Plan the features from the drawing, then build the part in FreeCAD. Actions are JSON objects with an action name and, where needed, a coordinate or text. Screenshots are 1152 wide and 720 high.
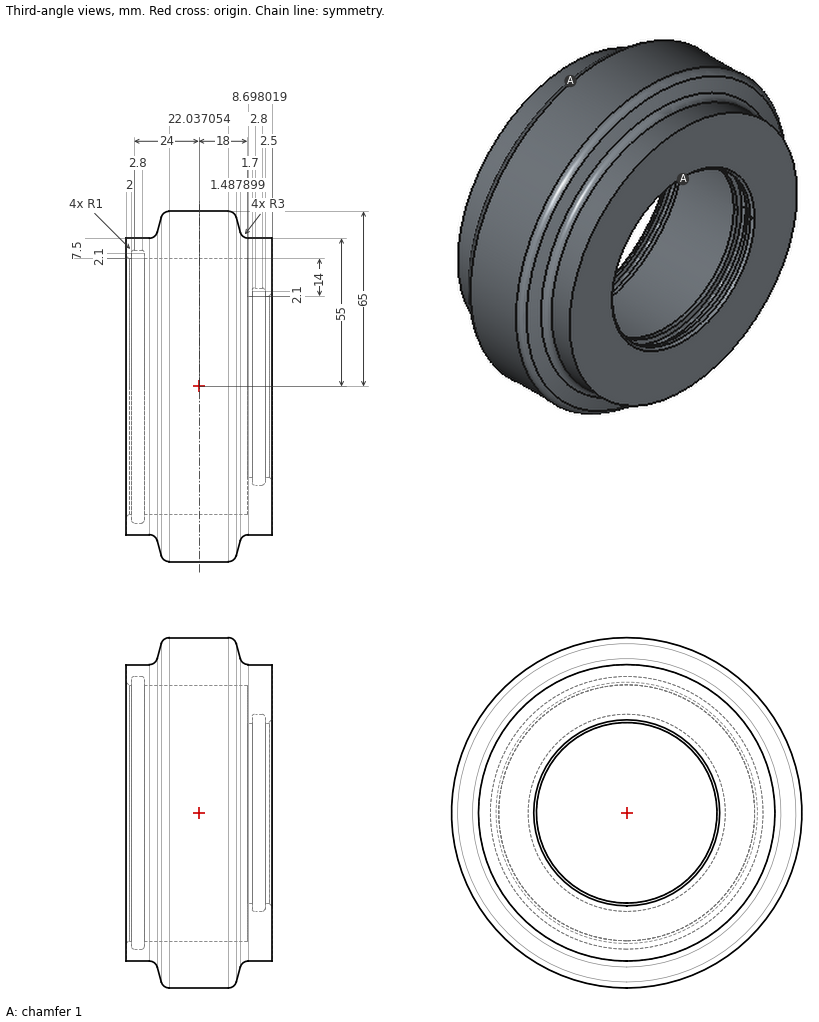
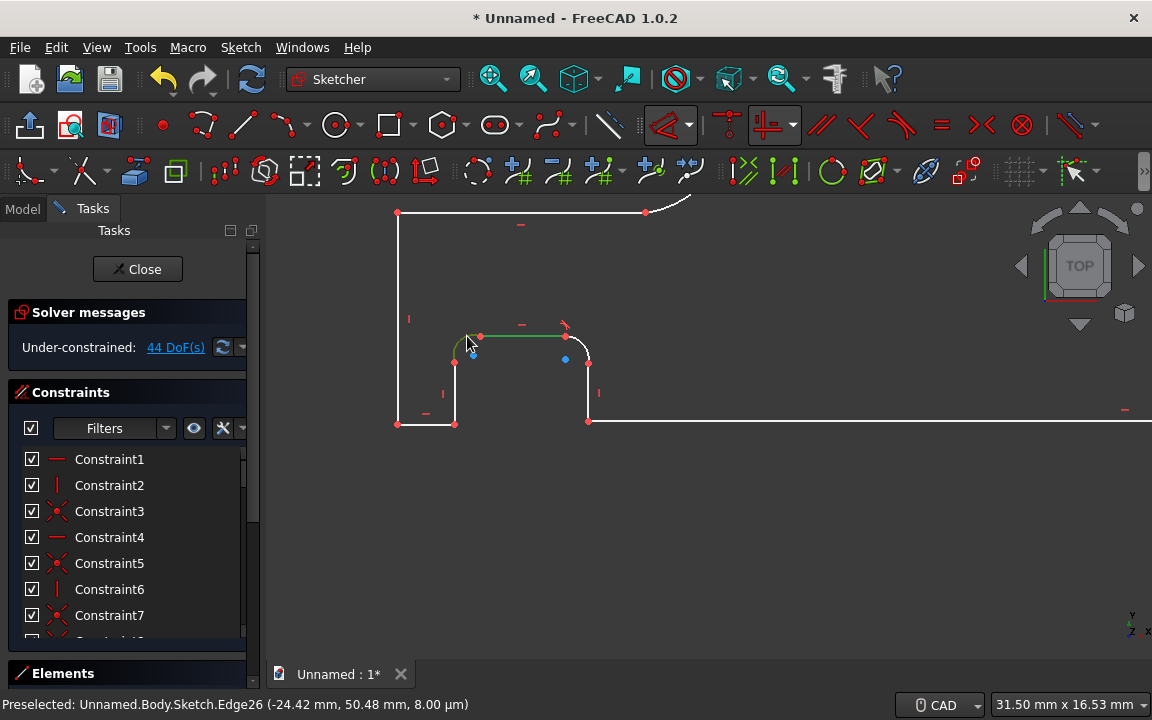
{"action": "left_click", "coordinate": [902, 126]}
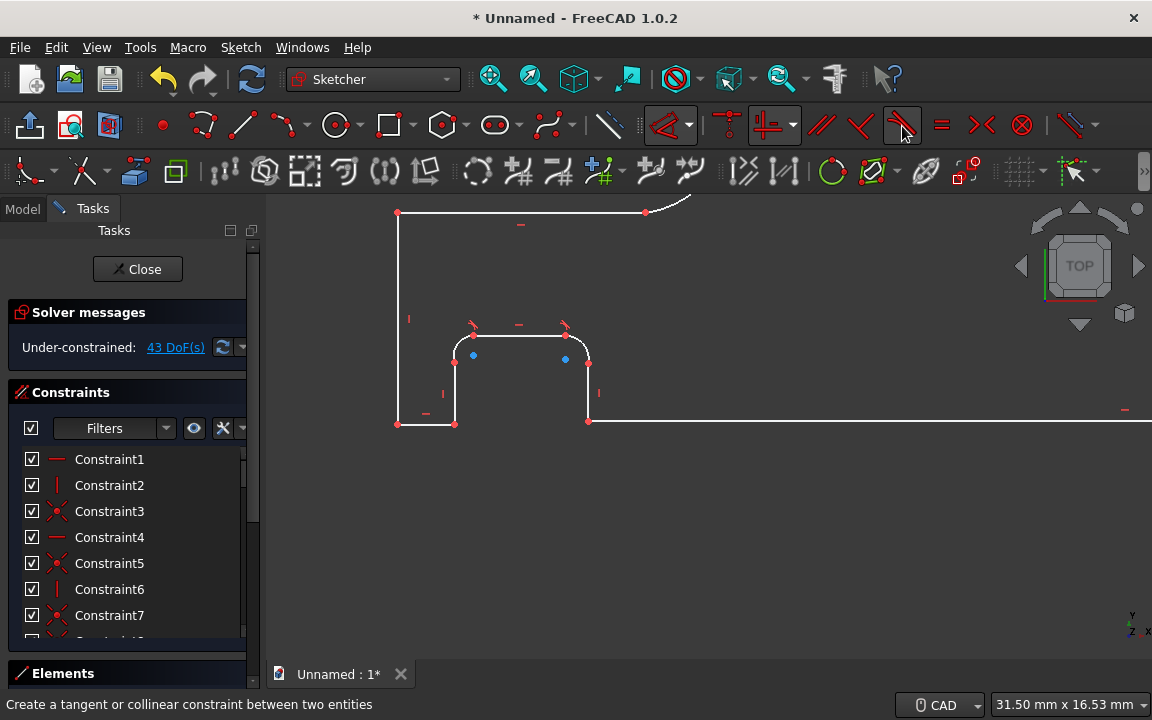
{"action": "left_click", "coordinate": [588, 381]}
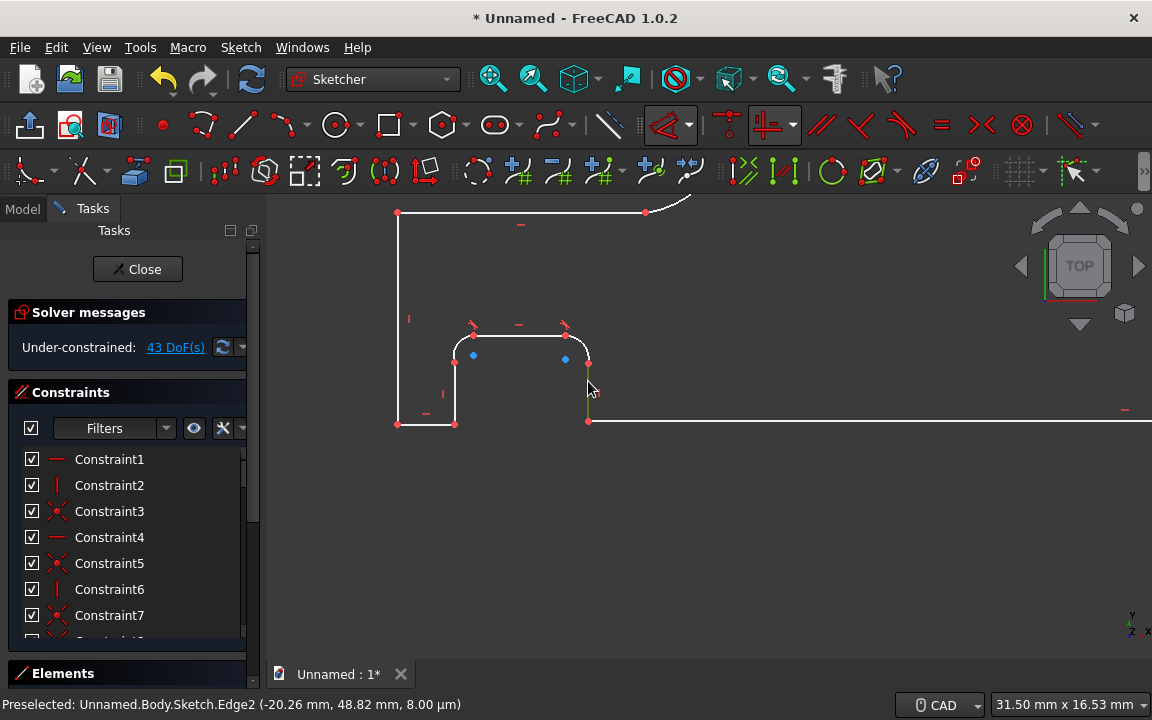
{"action": "left_click", "coordinate": [587, 352]}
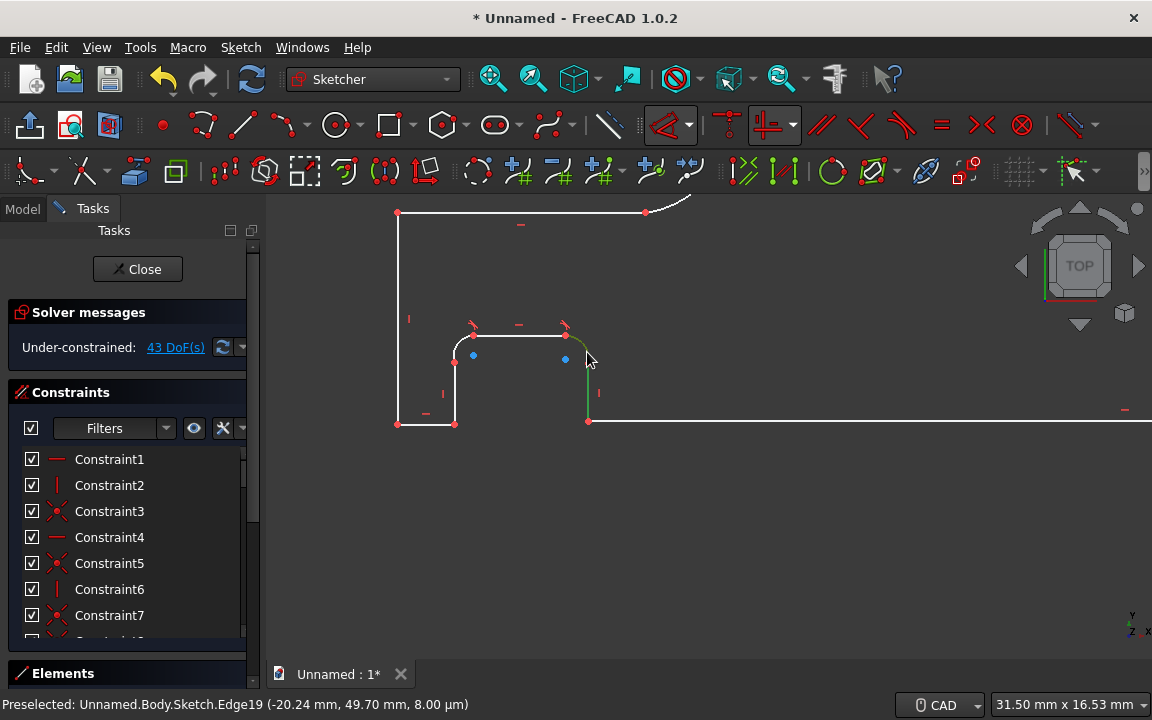
{"action": "key", "text": "t"}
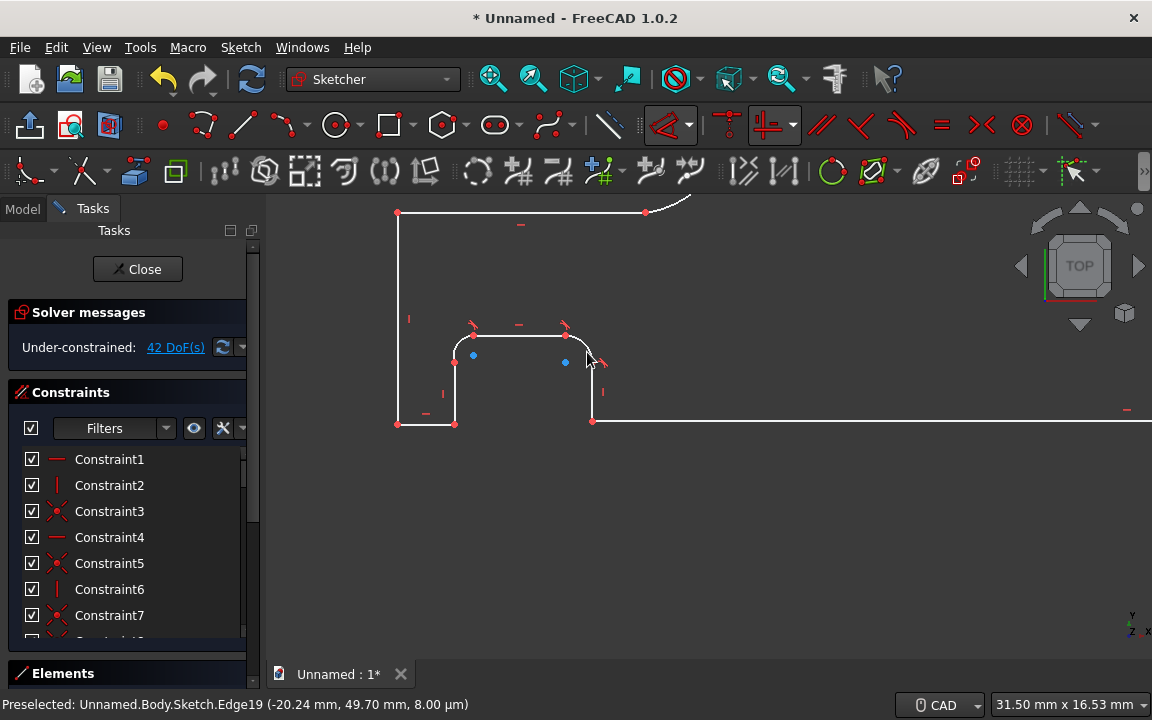
{"action": "scroll", "coordinate": [538, 344], "scroll_direction": "down", "scroll_amount": 9}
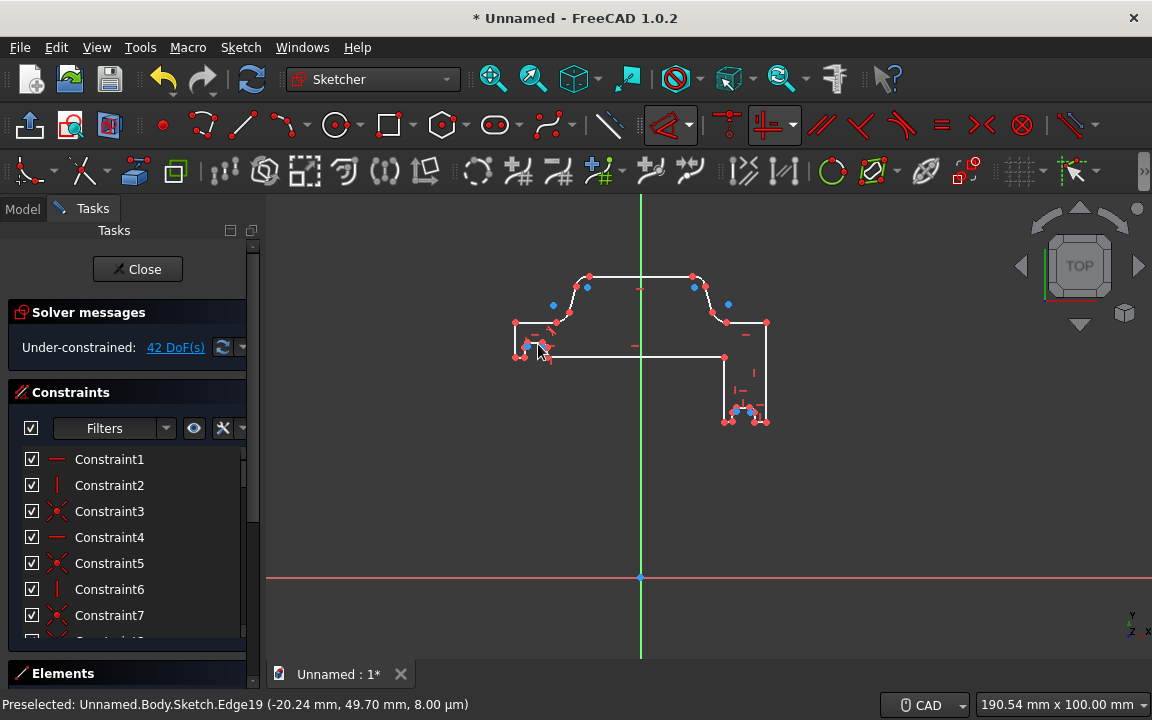
{"action": "scroll", "coordinate": [732, 419], "scroll_direction": "up", "scroll_amount": 8}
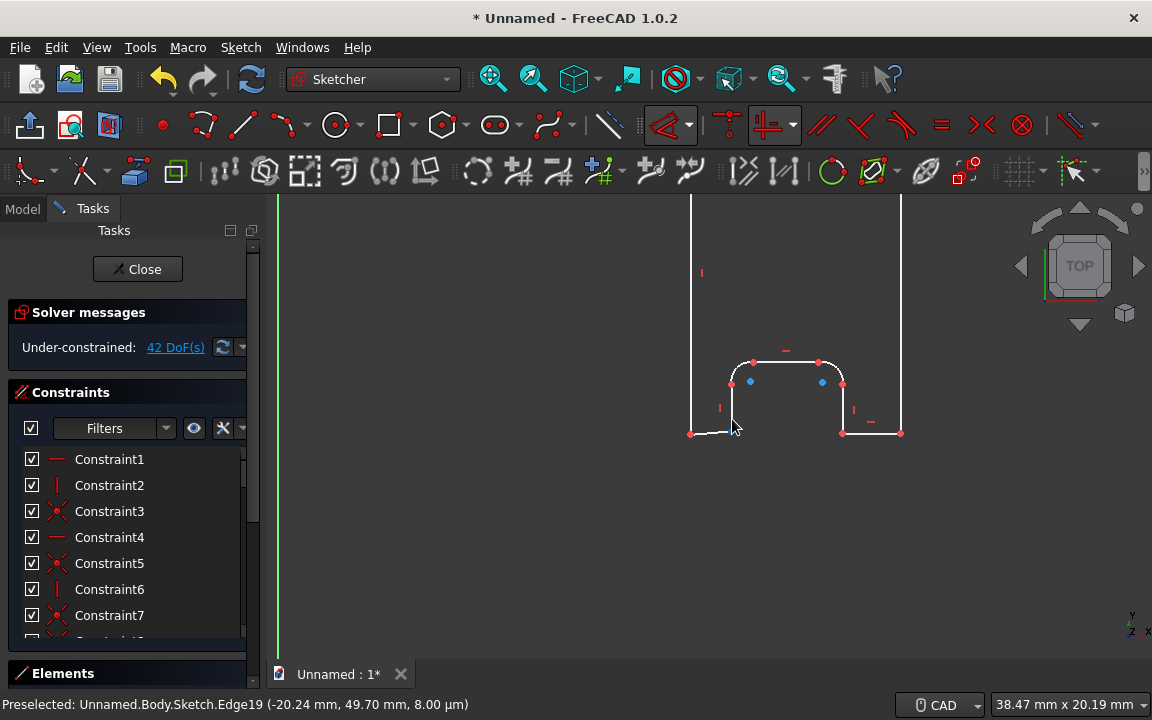
{"action": "left_click", "coordinate": [732, 417]}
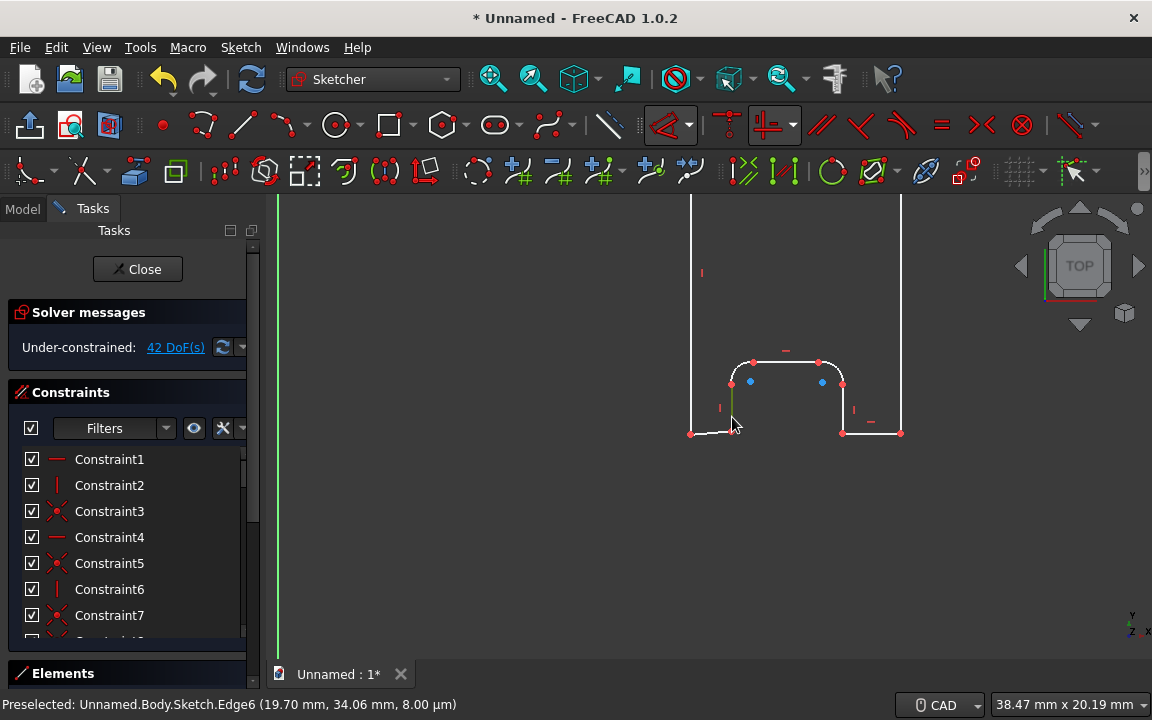
{"action": "scroll", "coordinate": [743, 364], "scroll_direction": "up", "scroll_amount": 2}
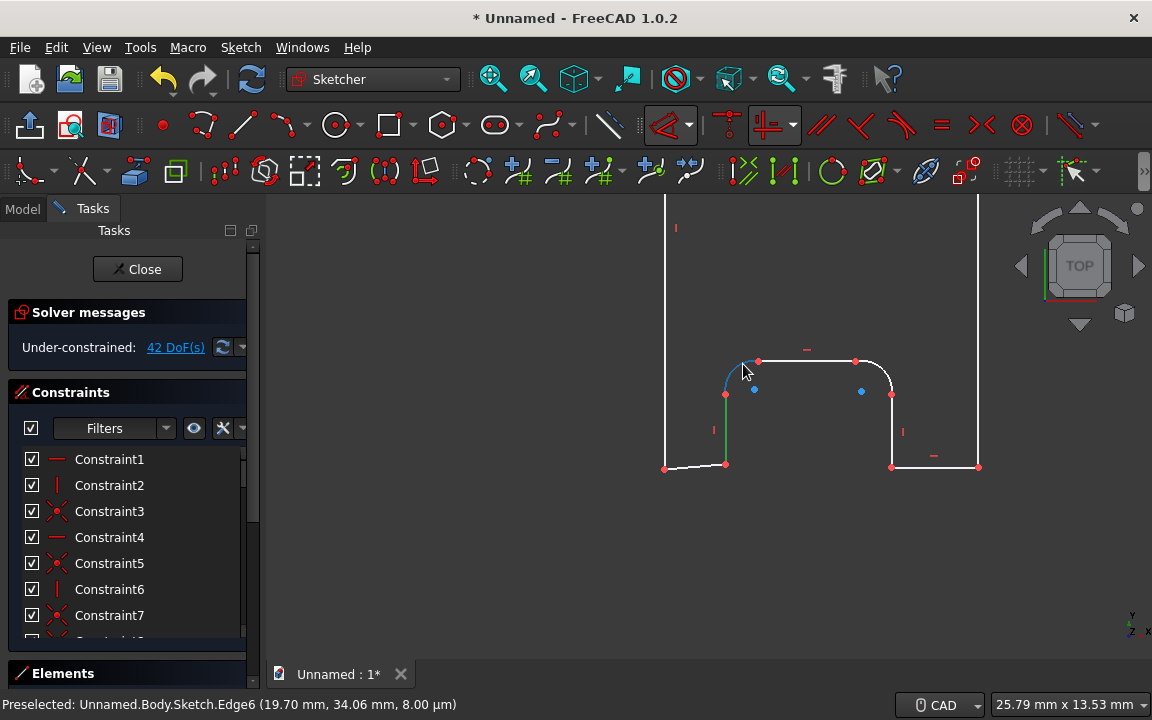
{"action": "left_click", "coordinate": [743, 363]}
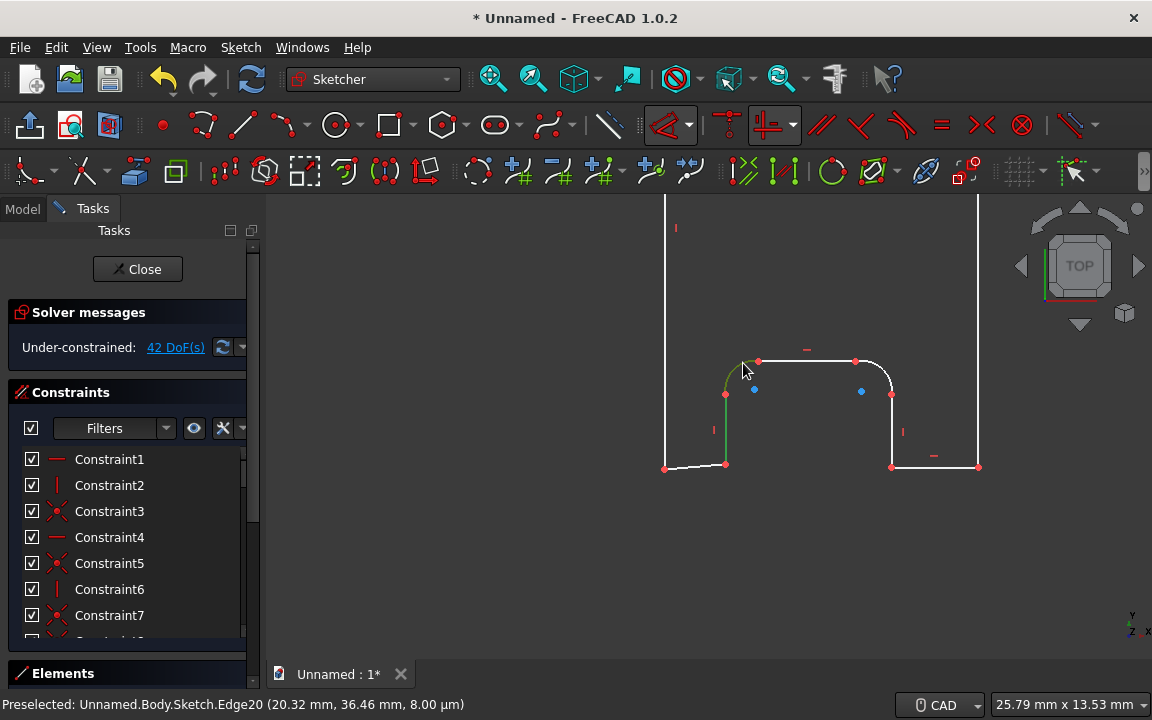
{"action": "key", "text": "t"}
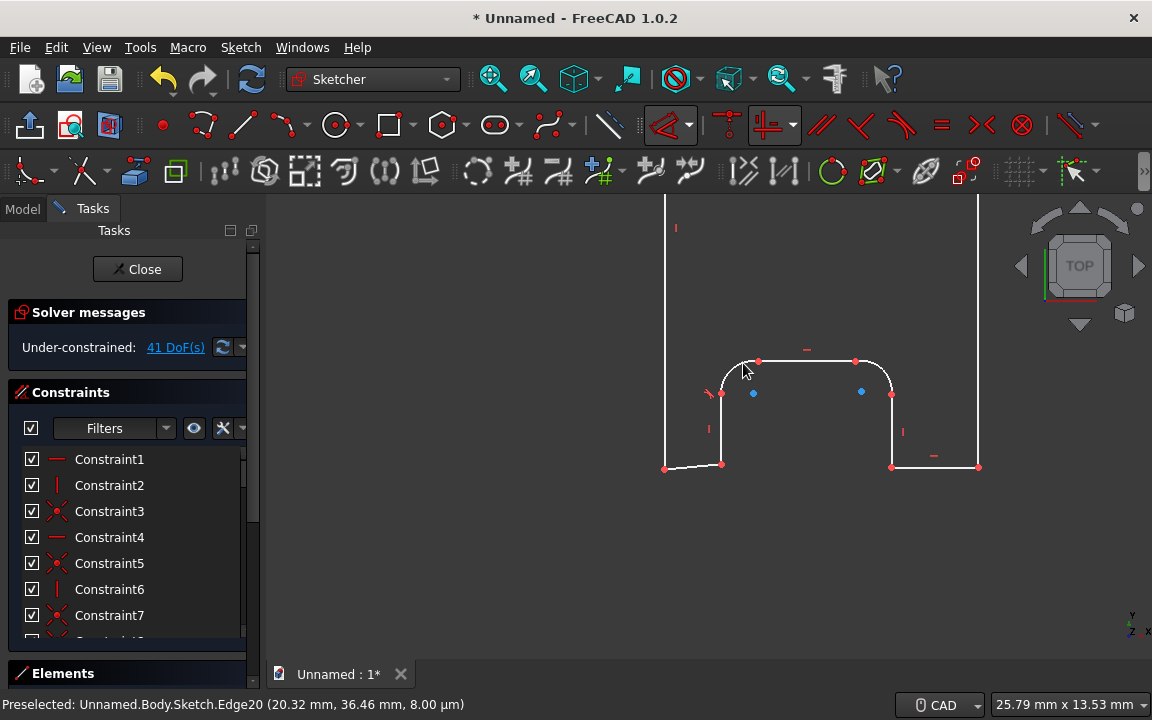
{"action": "left_click", "coordinate": [788, 361]}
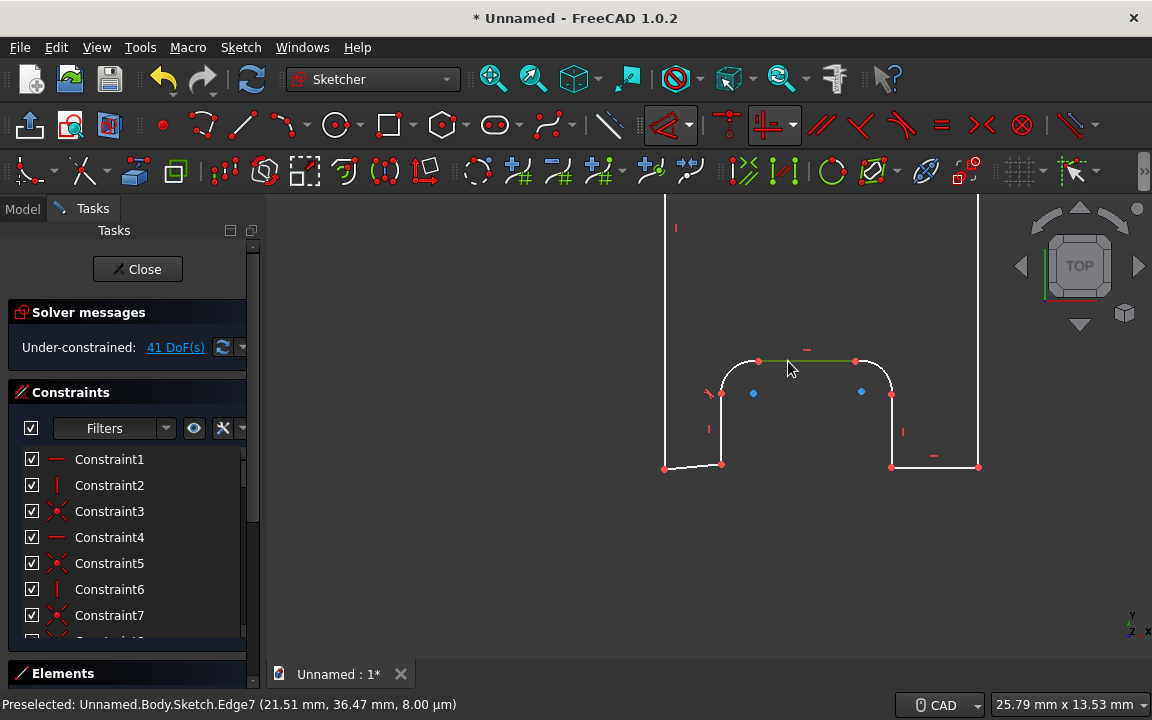
{"action": "left_click", "coordinate": [742, 363]}